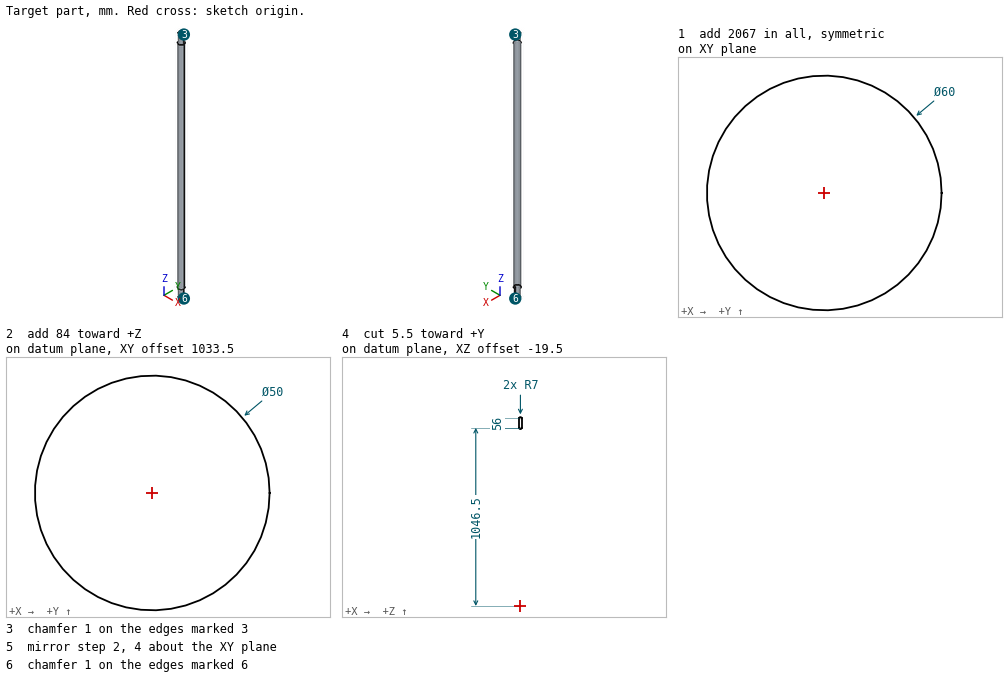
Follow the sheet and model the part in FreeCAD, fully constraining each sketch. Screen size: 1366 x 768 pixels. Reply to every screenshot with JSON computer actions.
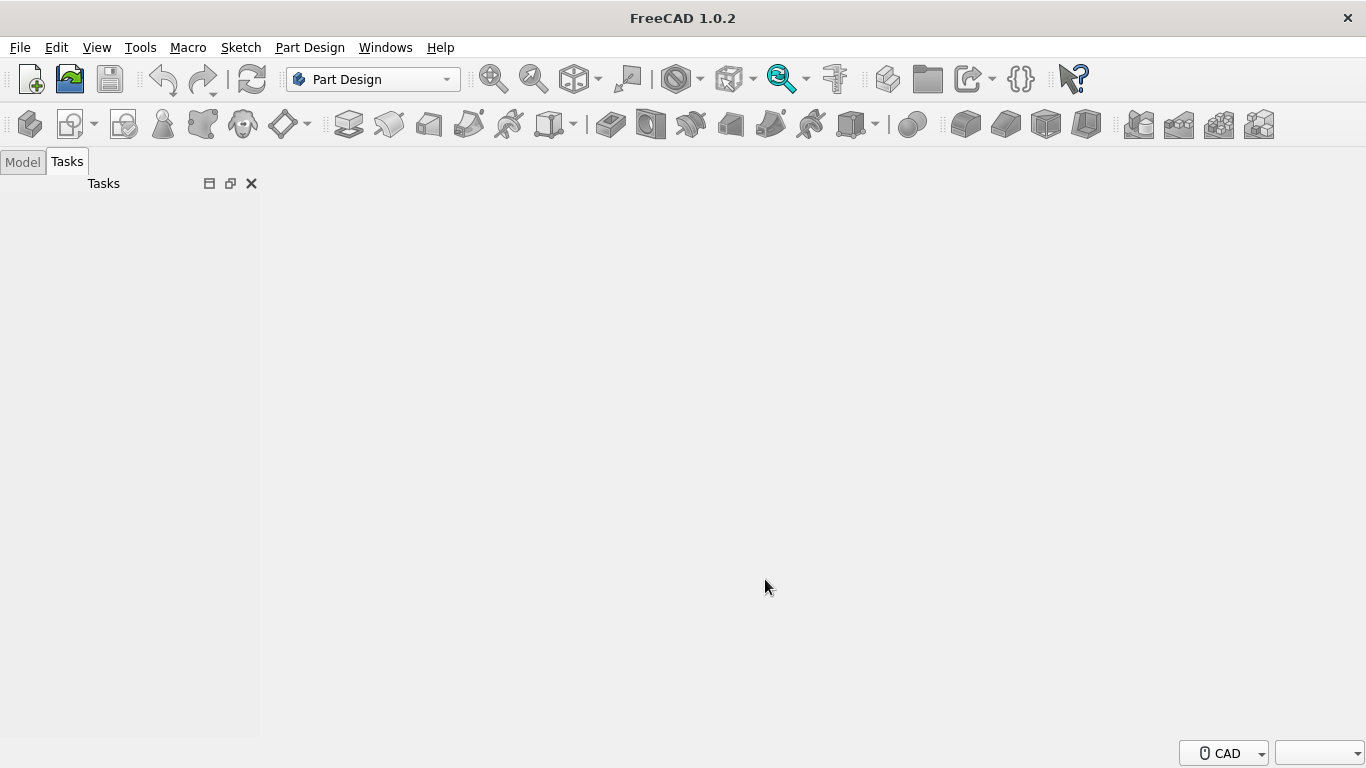
{"action": "left_click", "coordinate": [30, 80]}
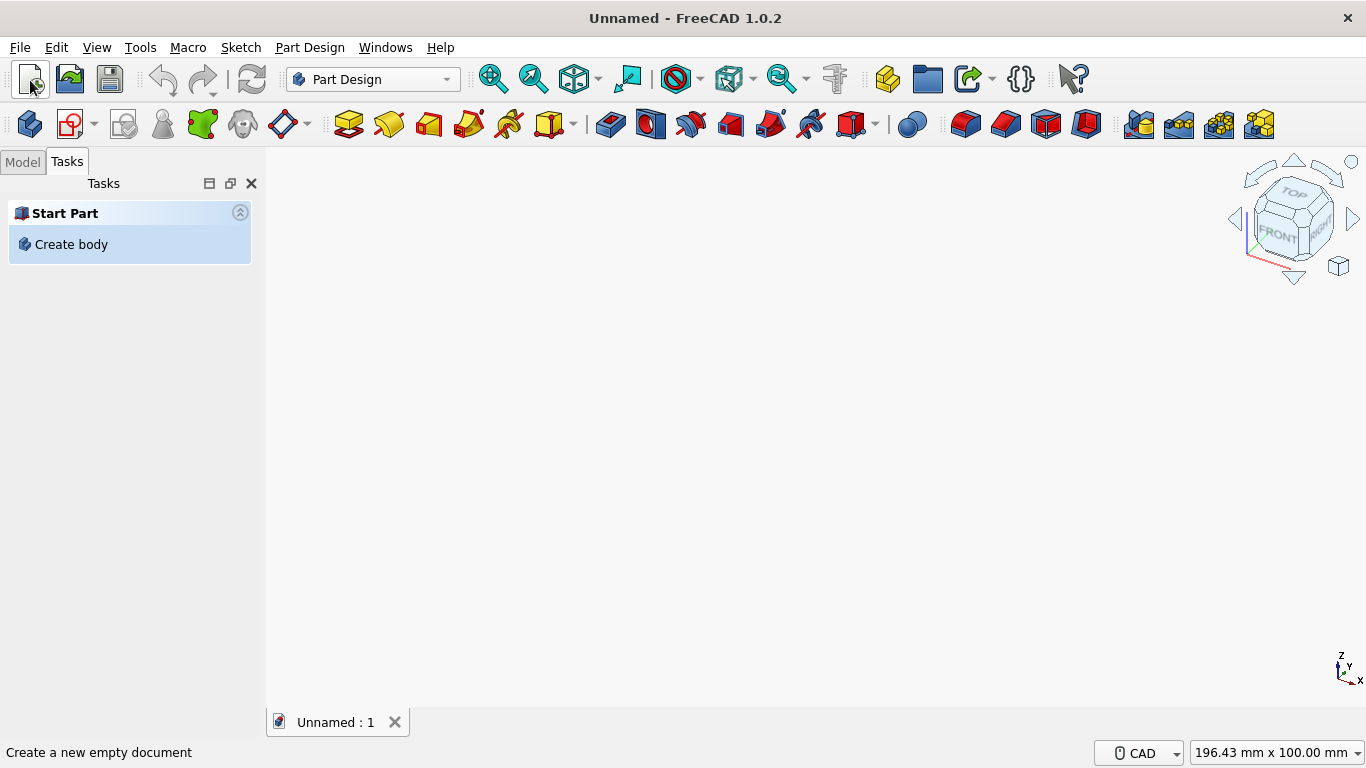
{"action": "left_click", "coordinate": [70, 124]}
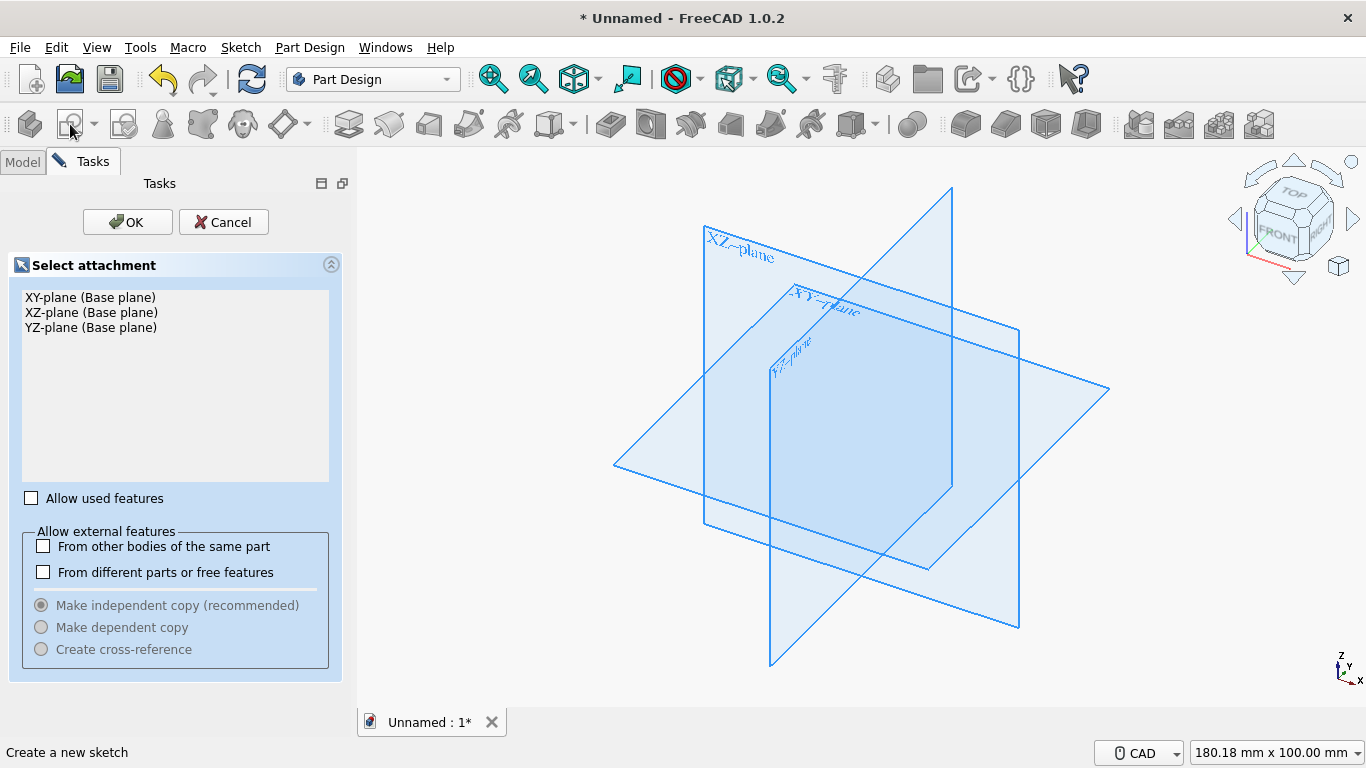
{"action": "left_click", "coordinate": [82, 298]}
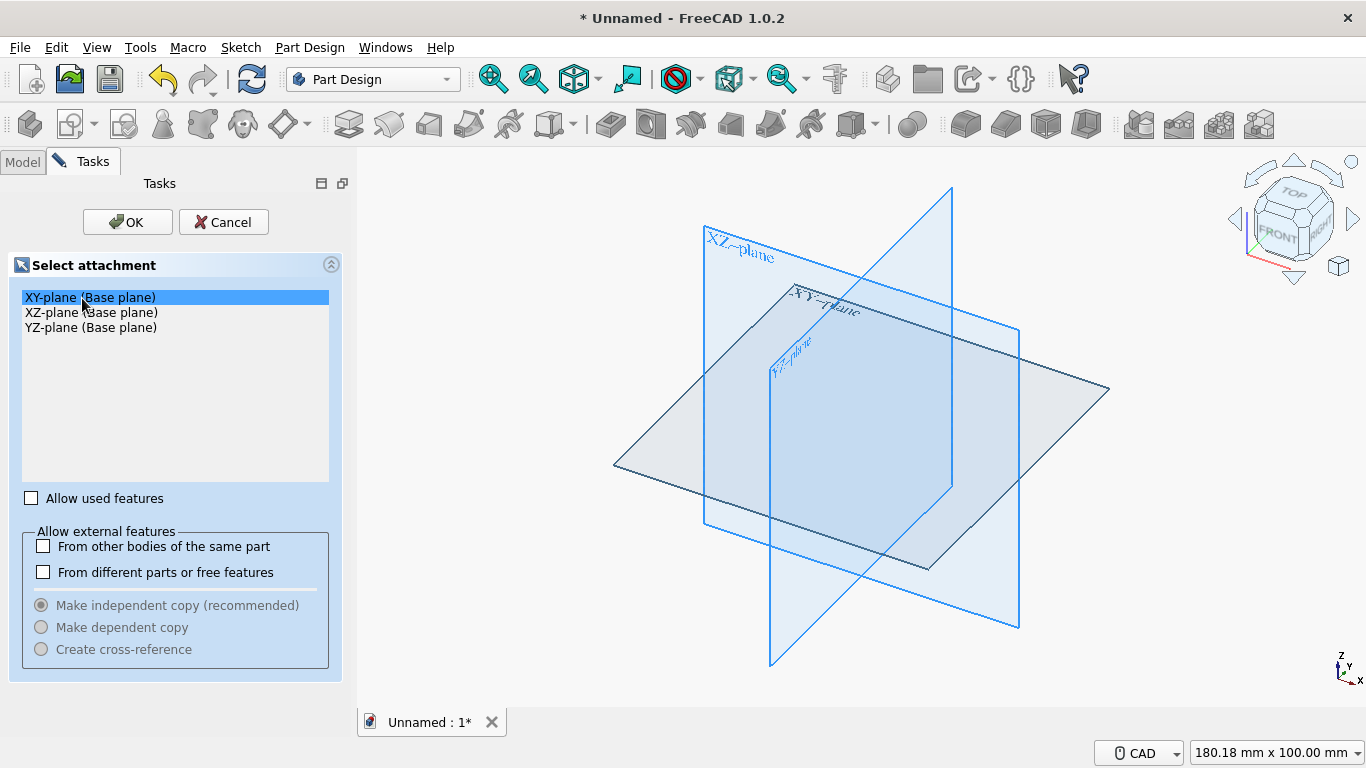
{"action": "left_click", "coordinate": [128, 222]}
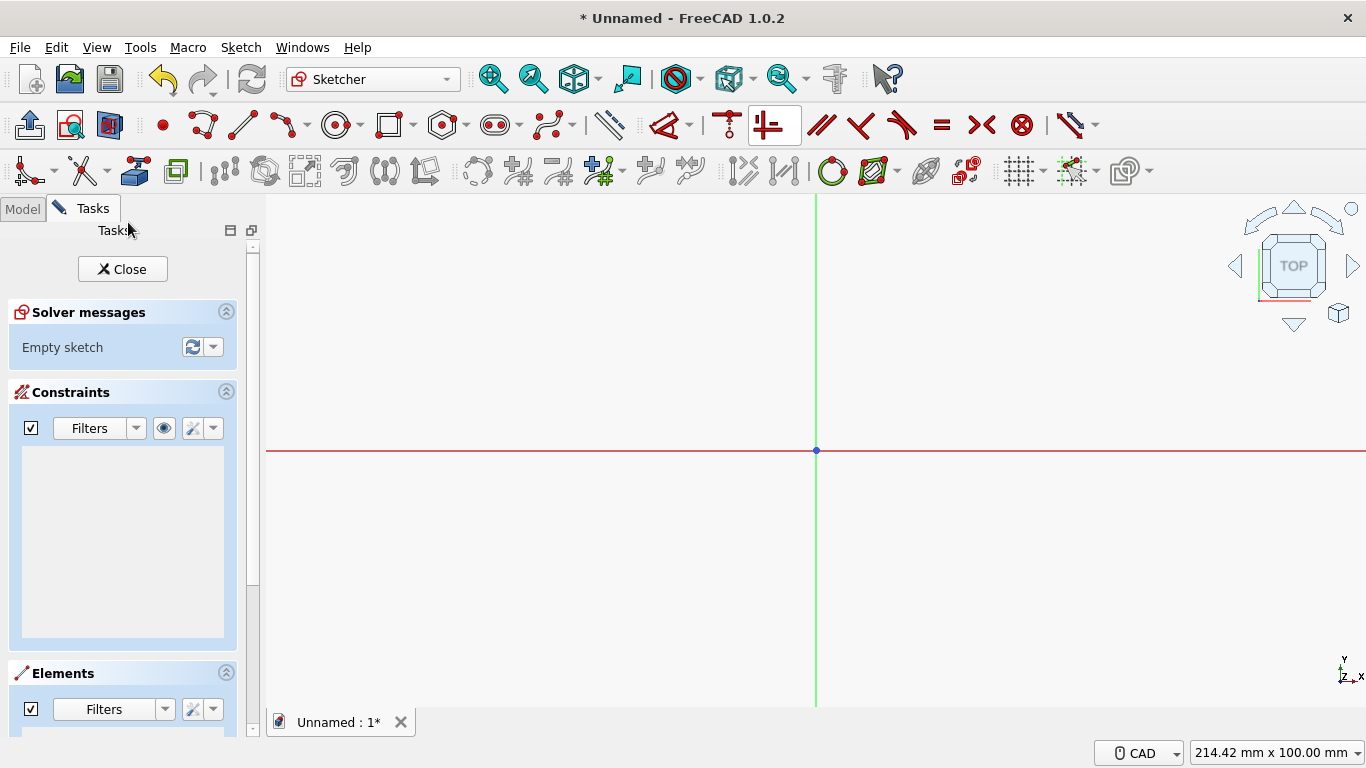
{"action": "left_click", "coordinate": [336, 126]}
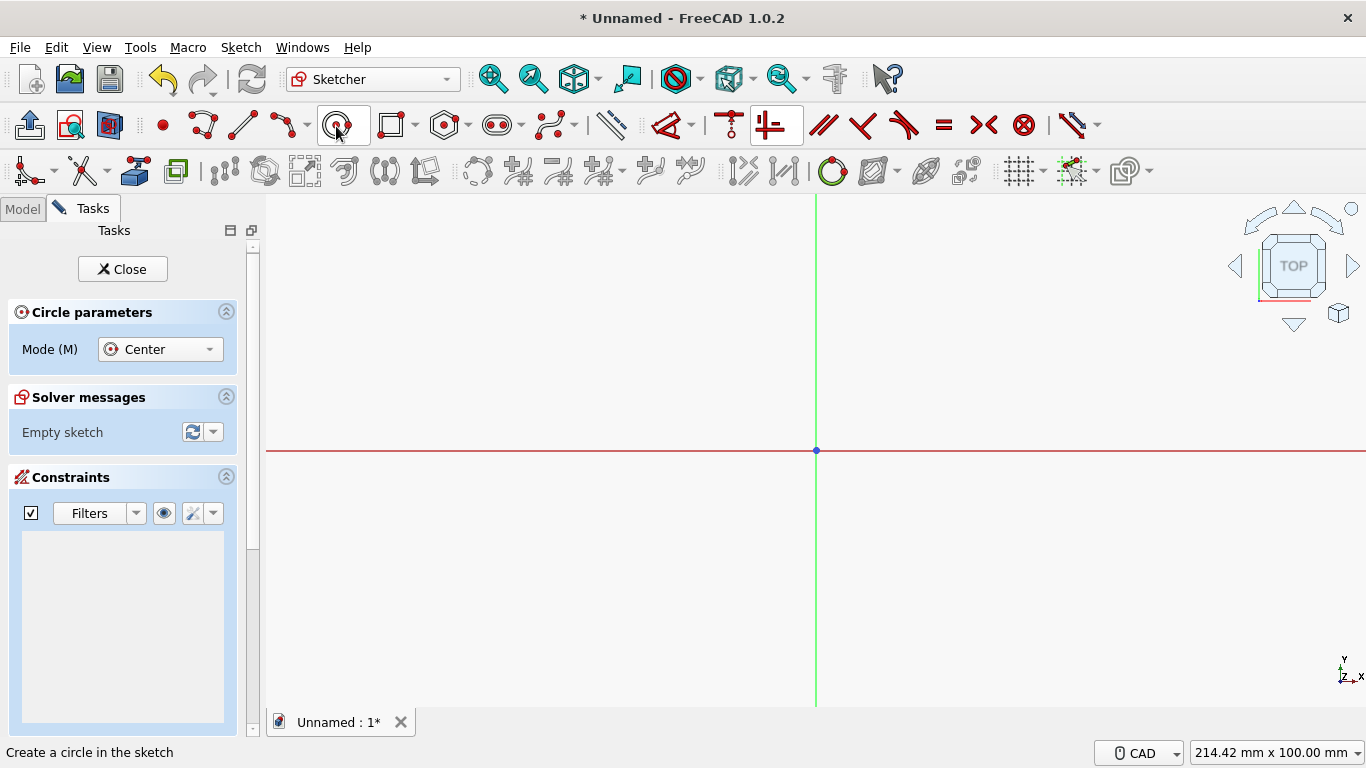
{"action": "left_click", "coordinate": [816, 450]}
{"action": "mouse_move", "coordinate": [925, 342]}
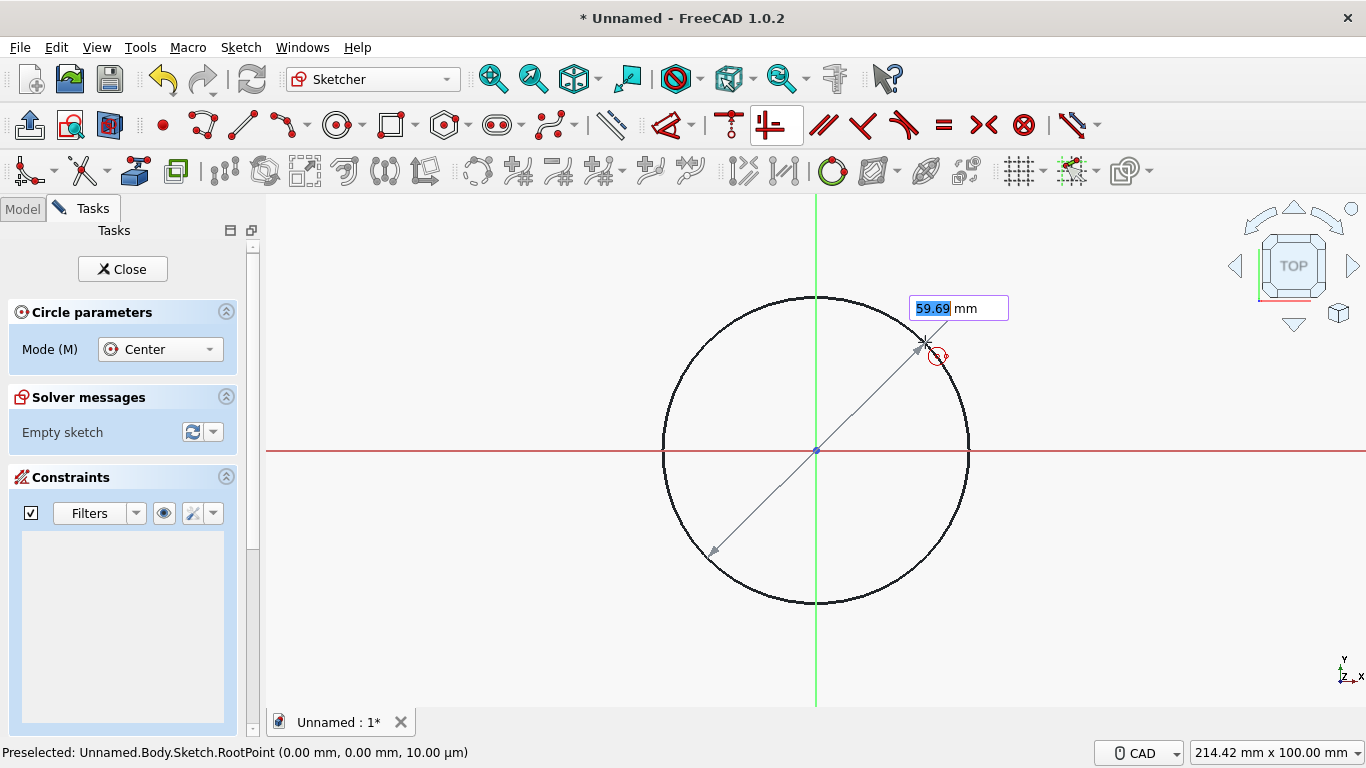
{"action": "type", "text": "60"}
{"action": "key", "text": "Return"}
{"action": "key", "text": "Escape"}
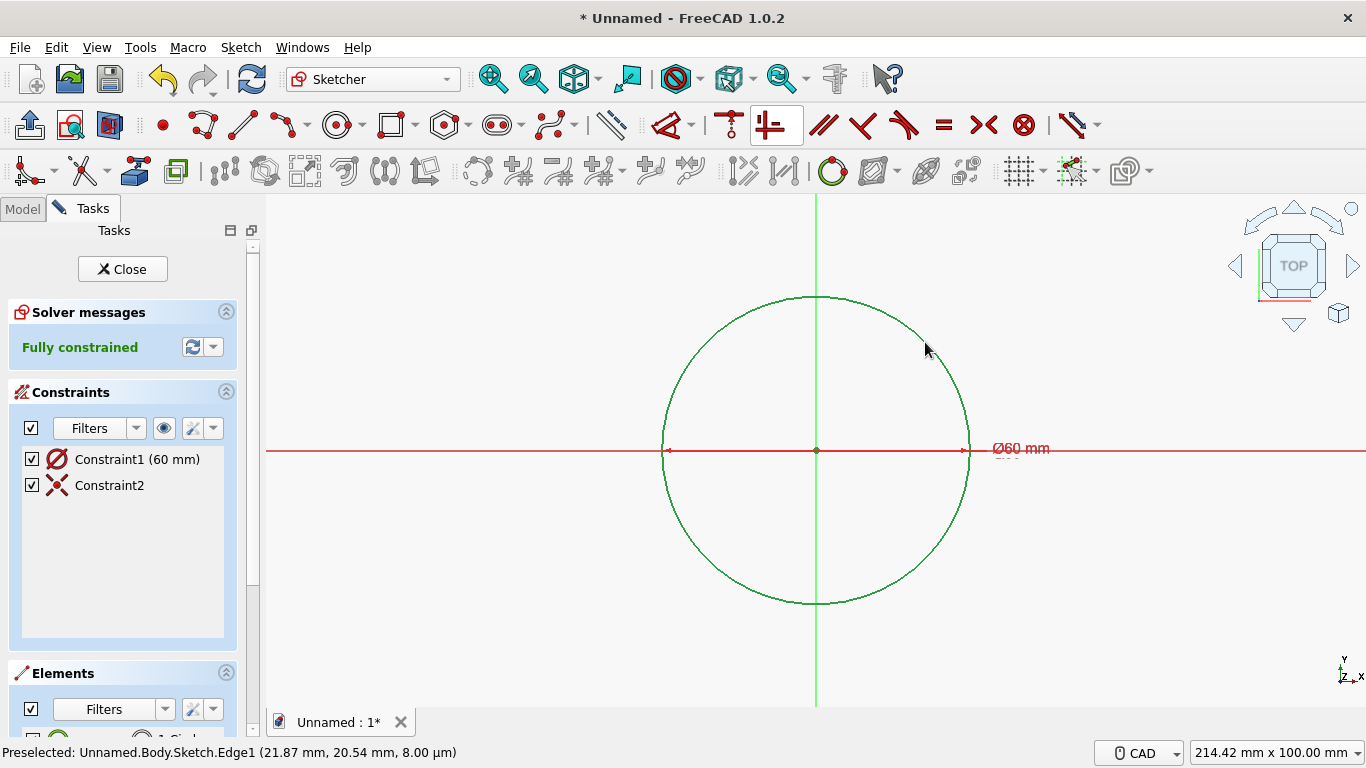
{"action": "left_click", "coordinate": [123, 269]}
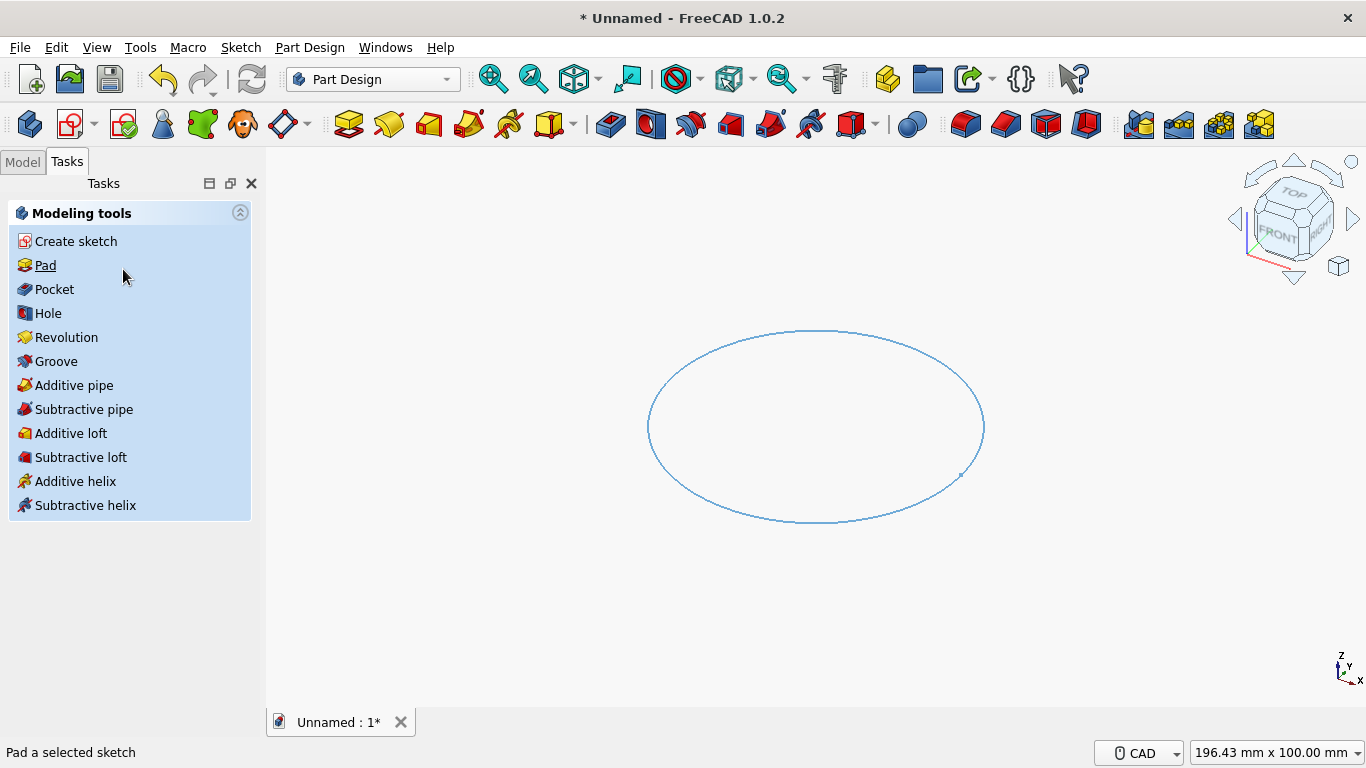
{"action": "left_click", "coordinate": [350, 124]}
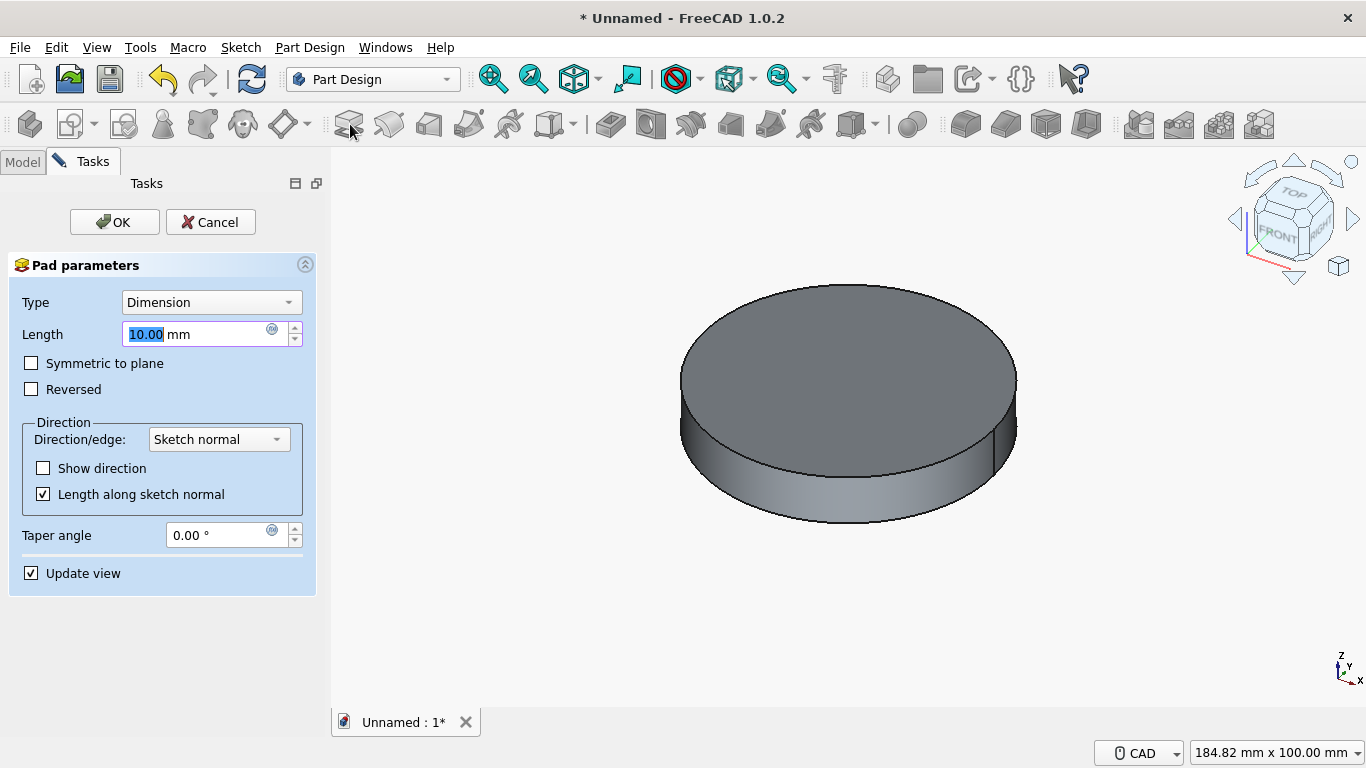
{"action": "type", "text": "2067"}
{"action": "key", "text": "Tab"}